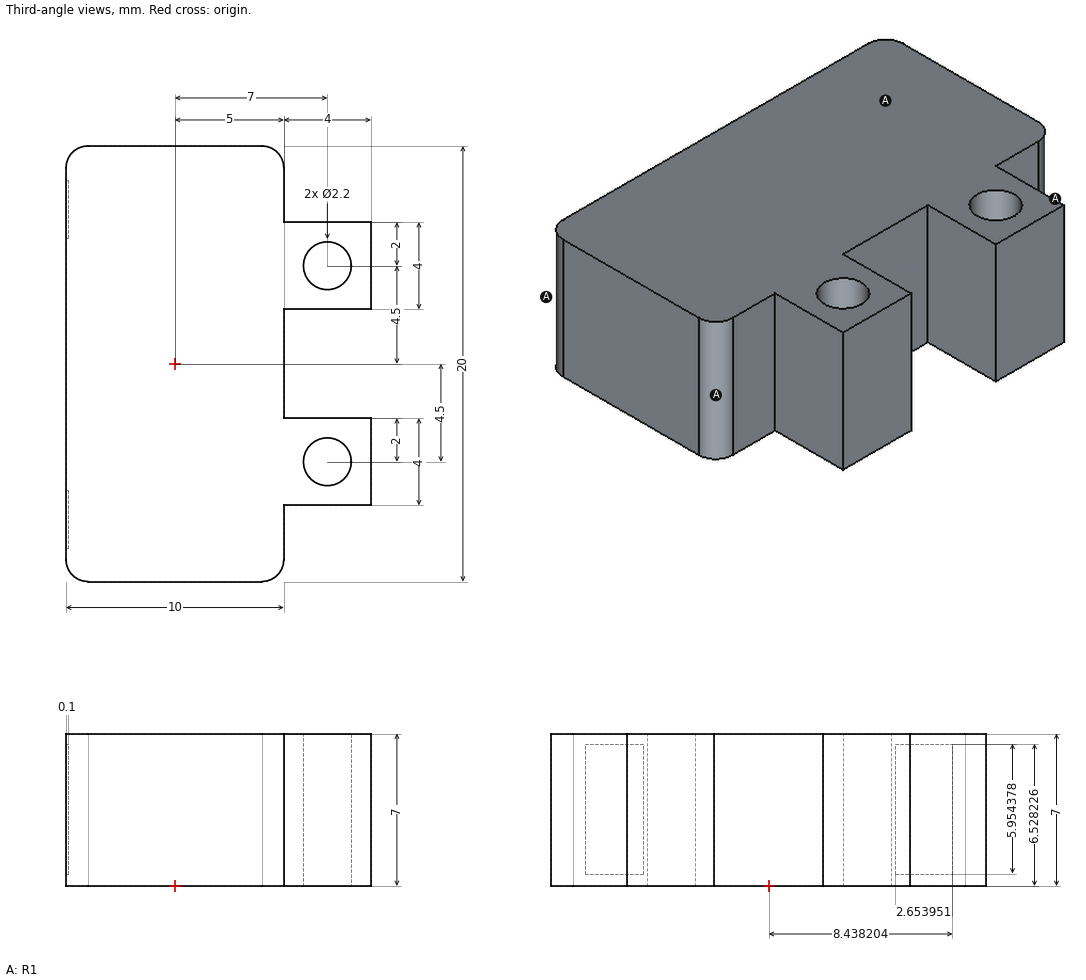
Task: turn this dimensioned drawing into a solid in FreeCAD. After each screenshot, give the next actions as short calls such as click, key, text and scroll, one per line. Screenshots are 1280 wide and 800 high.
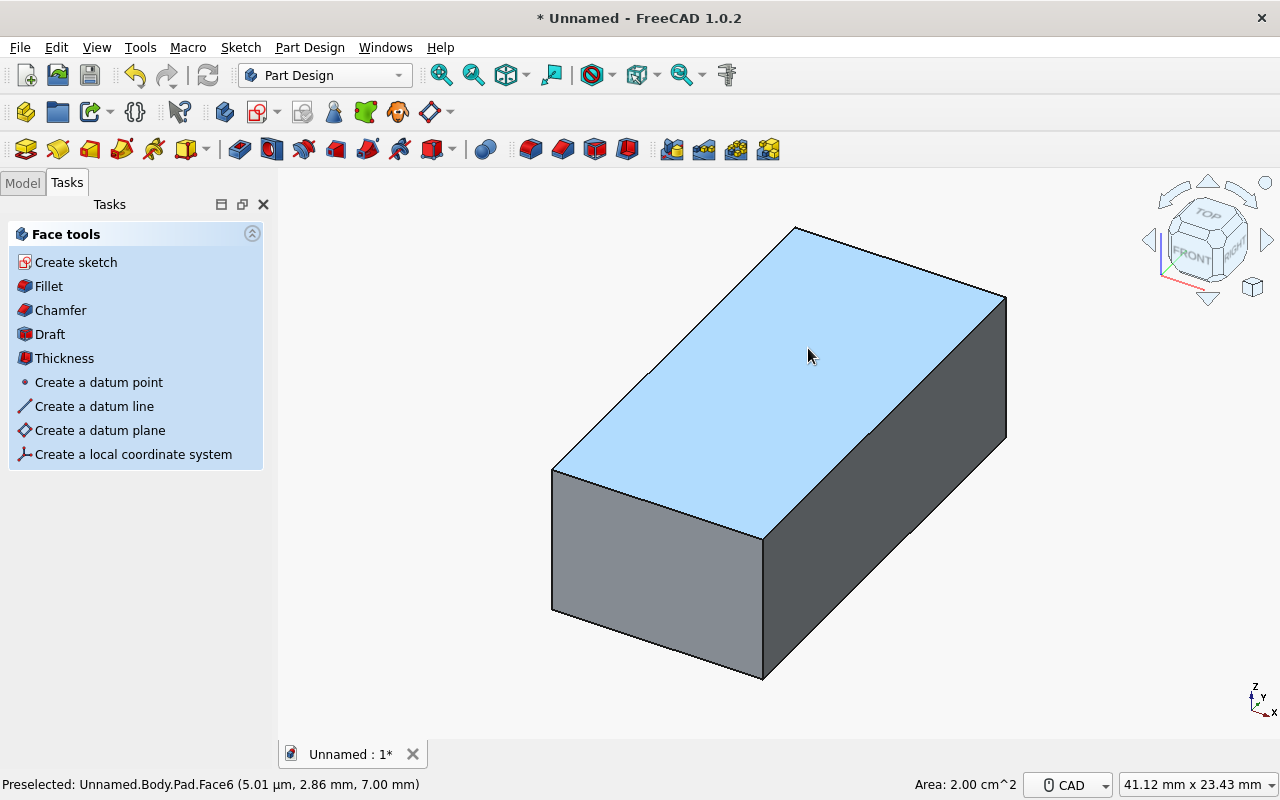
click(258, 112)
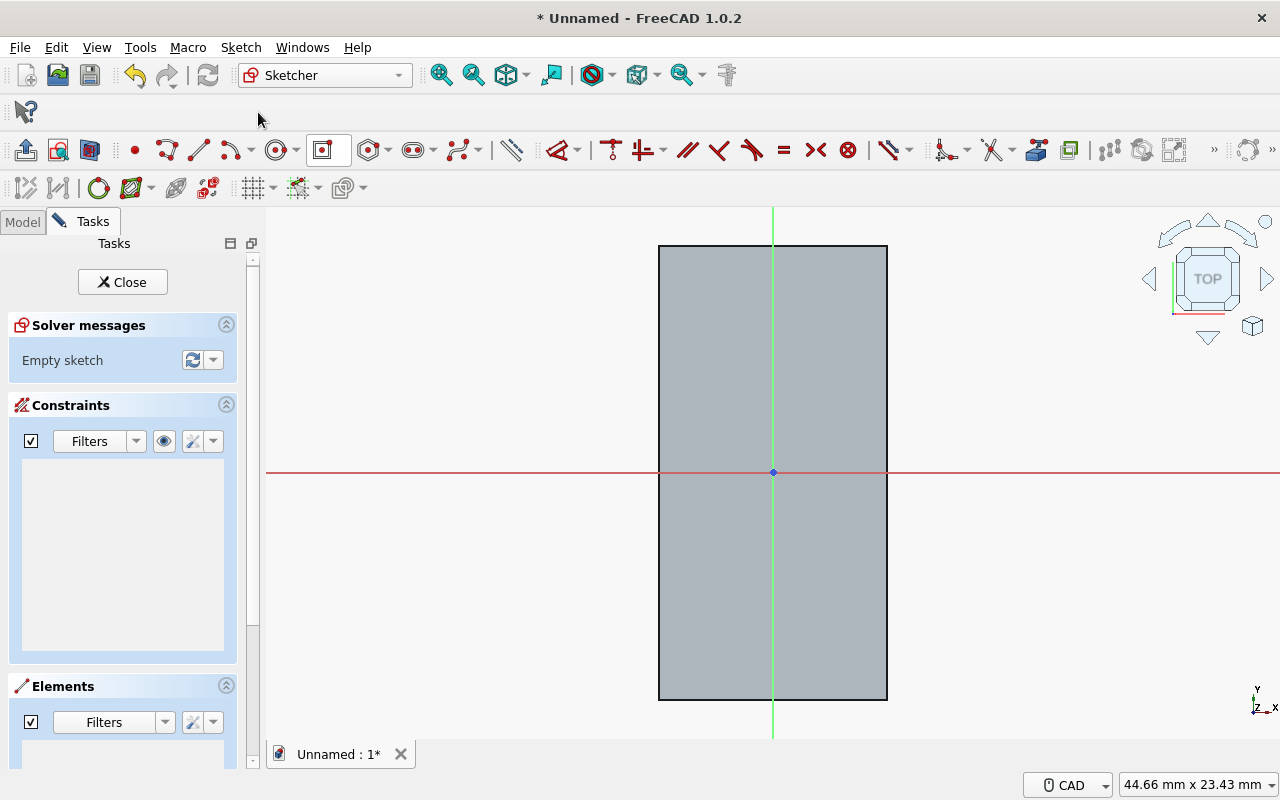
key(g)
key(r)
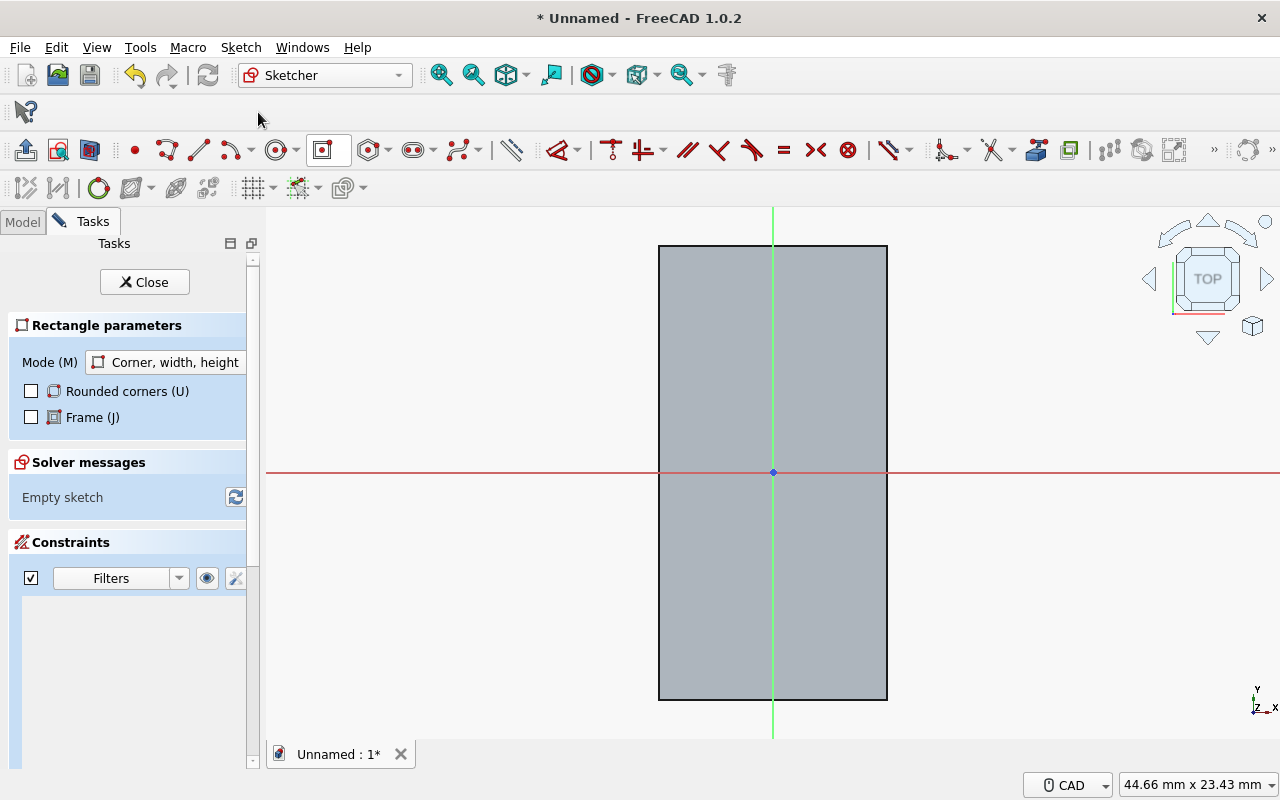
click(887, 325)
click(977, 416)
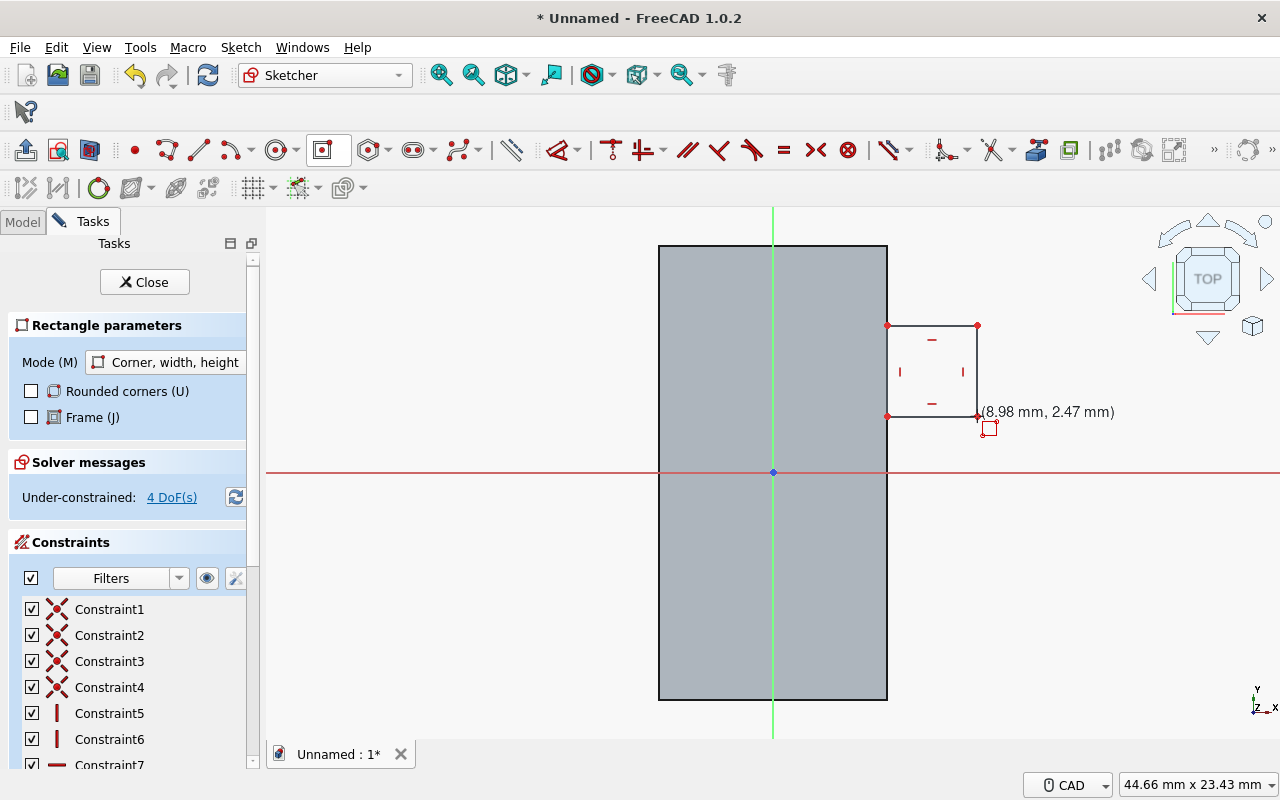
click(887, 530)
click(977, 621)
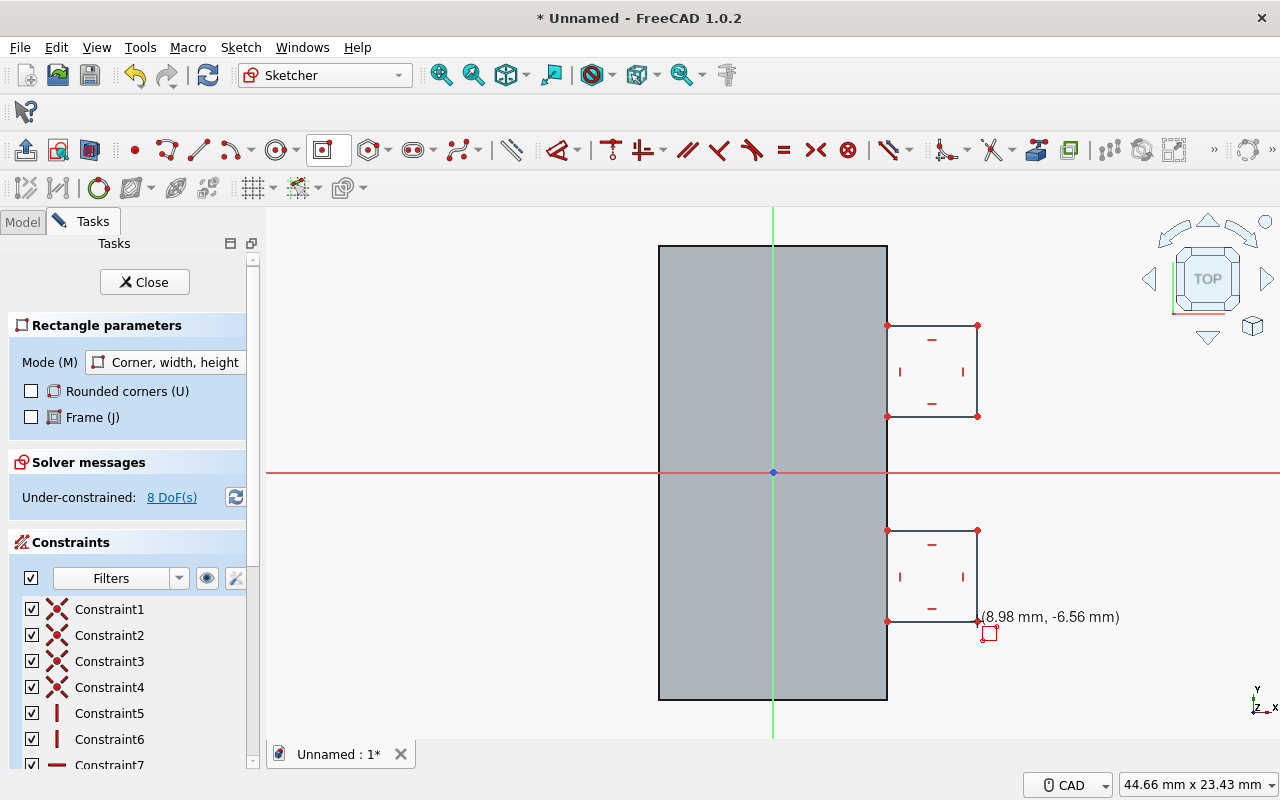
click(276, 150)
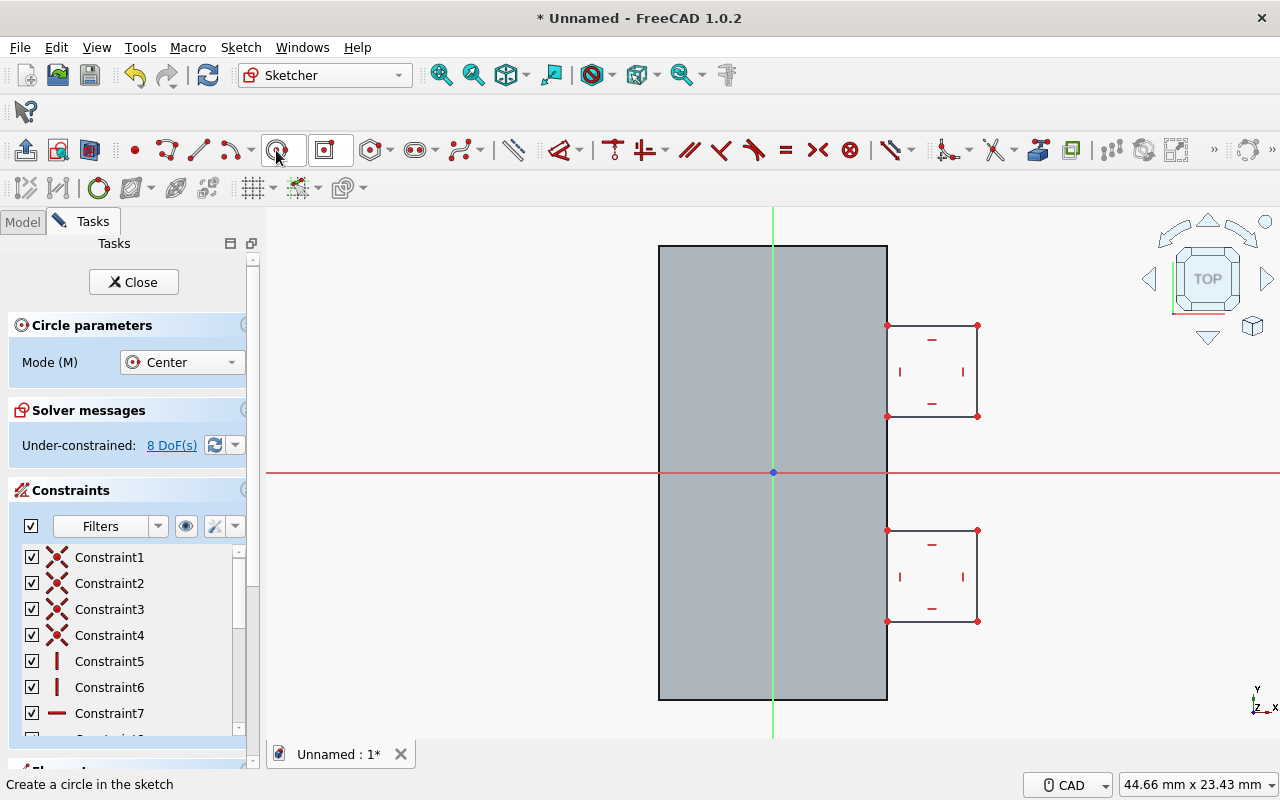
click(932, 371)
click(950, 353)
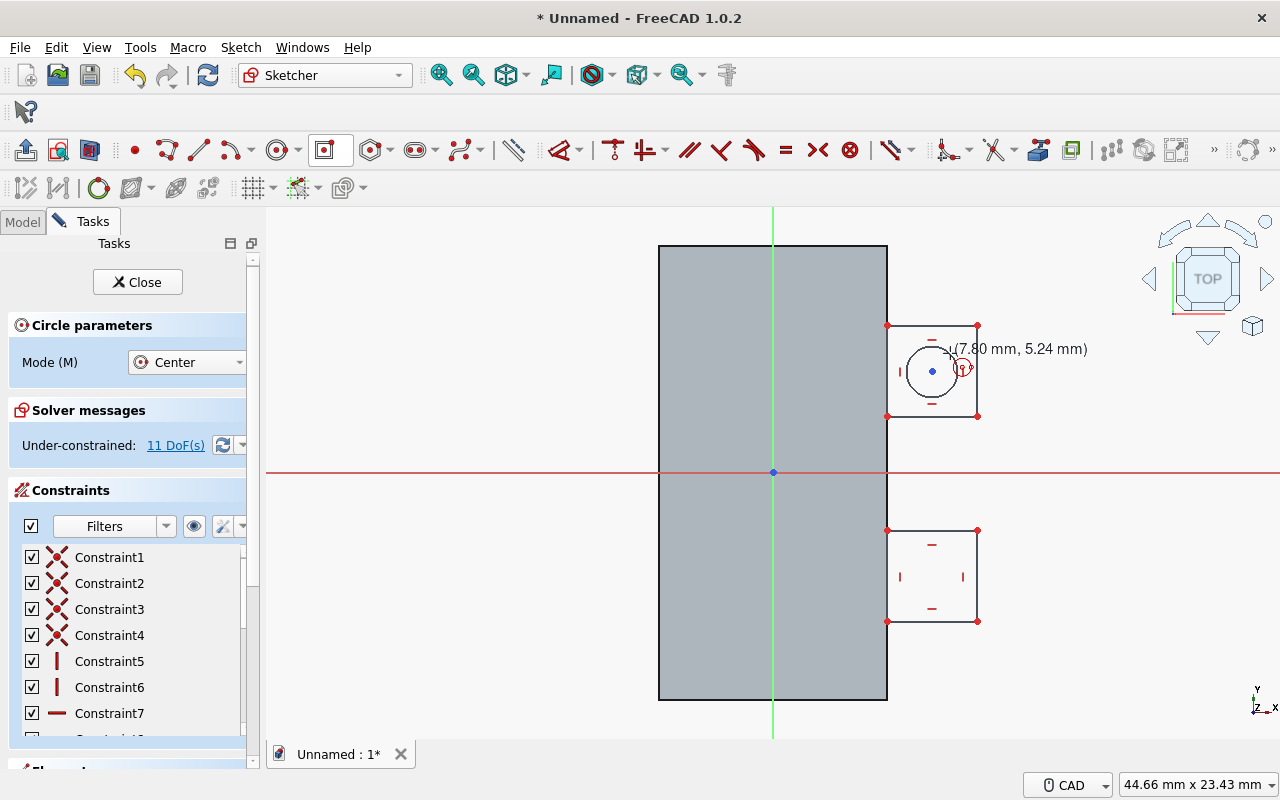
click(932, 575)
click(950, 558)
key(Escape)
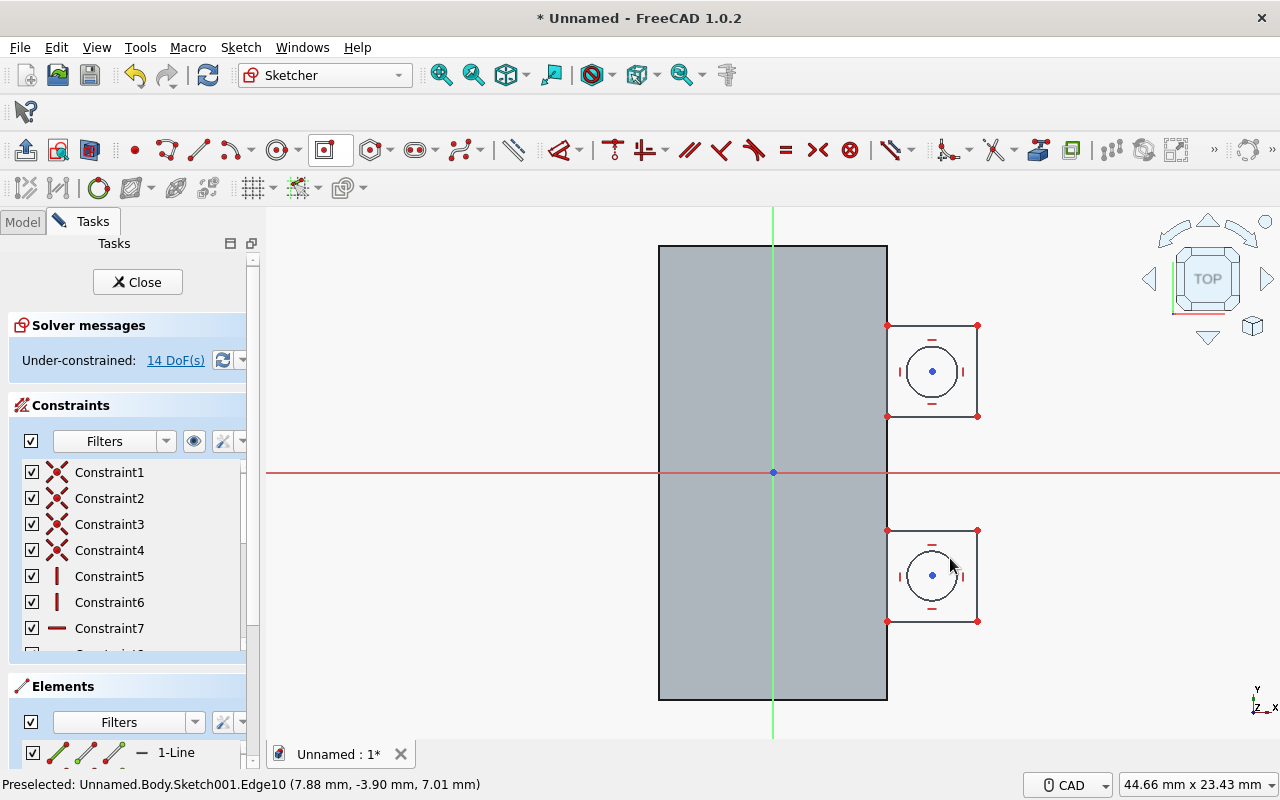
click(950, 354)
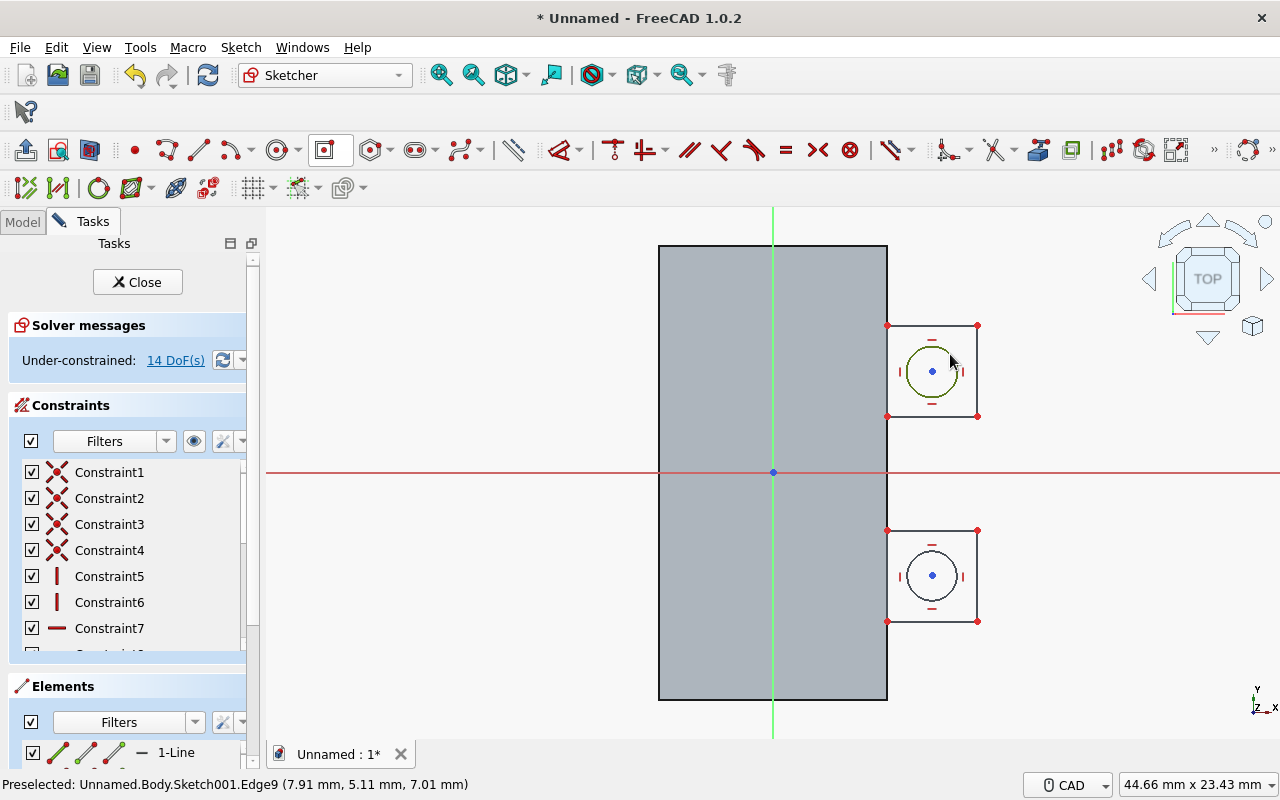
click(949, 558)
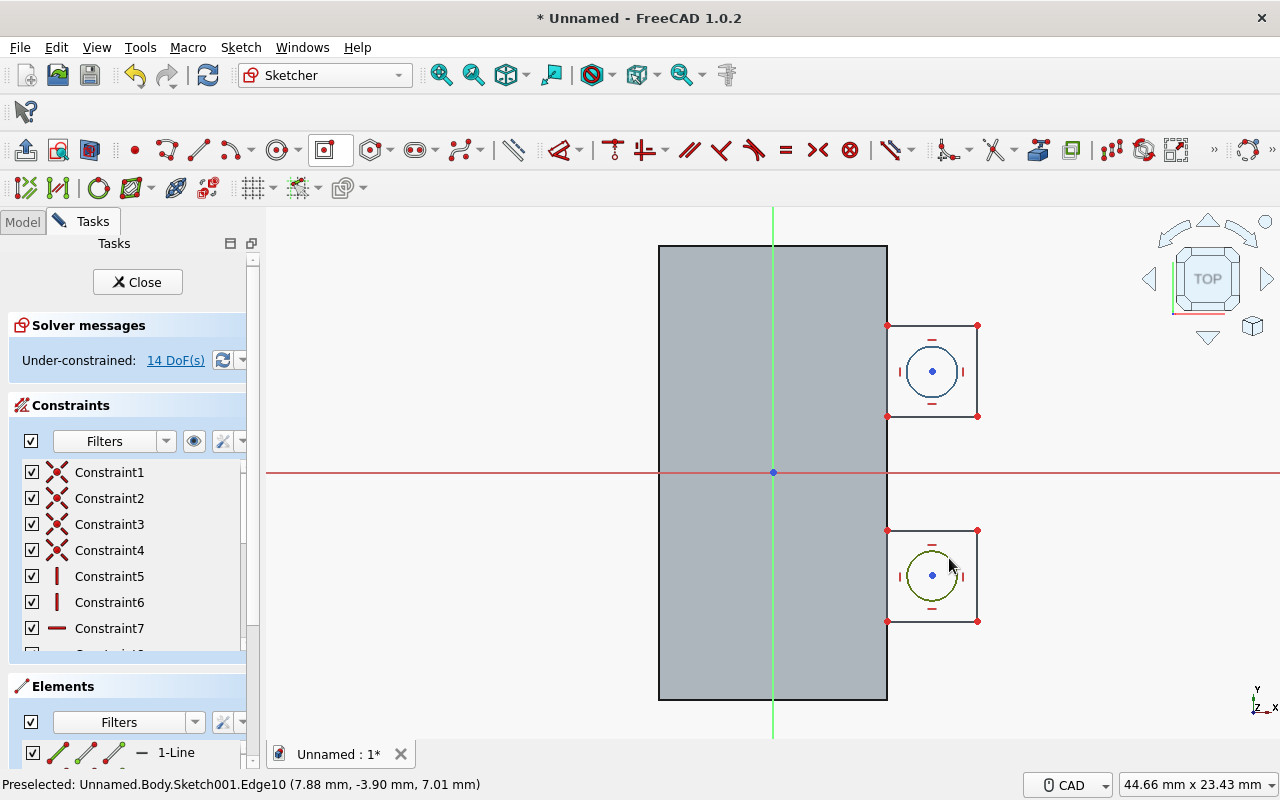
key(e)